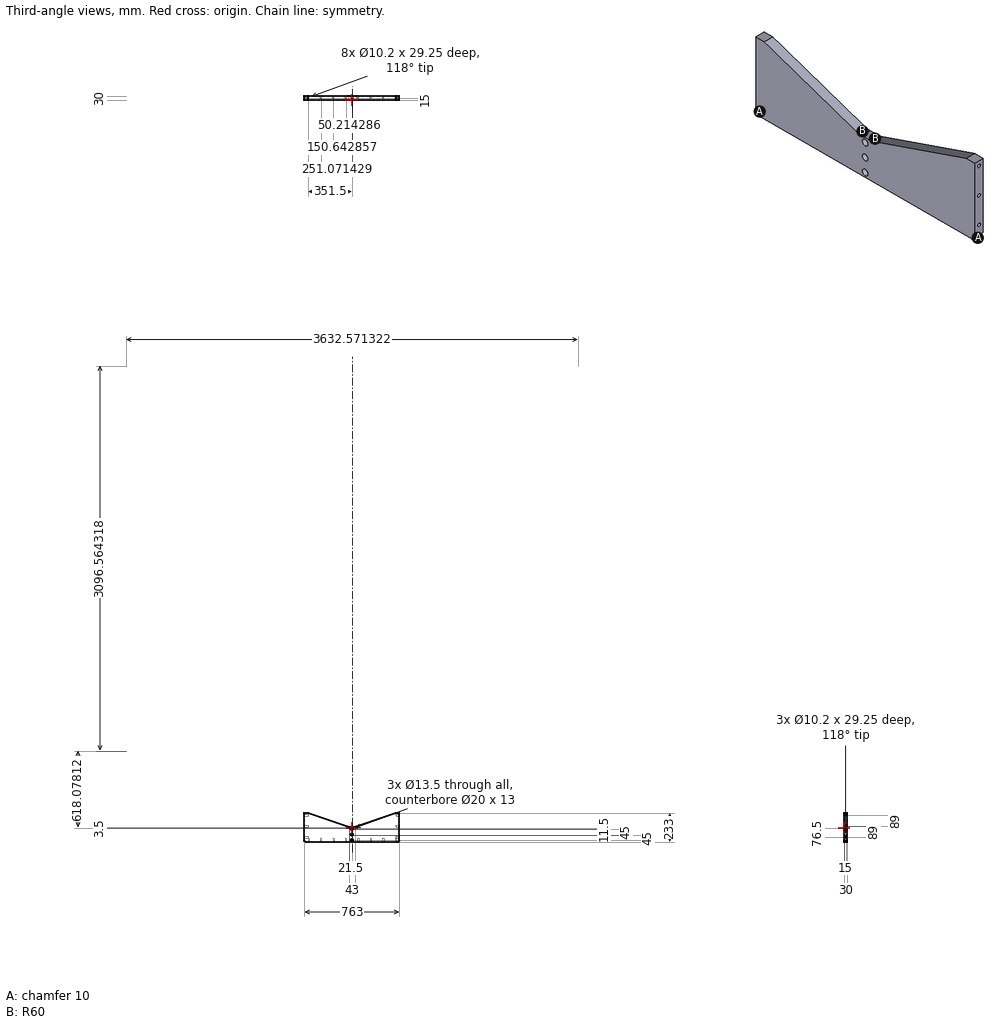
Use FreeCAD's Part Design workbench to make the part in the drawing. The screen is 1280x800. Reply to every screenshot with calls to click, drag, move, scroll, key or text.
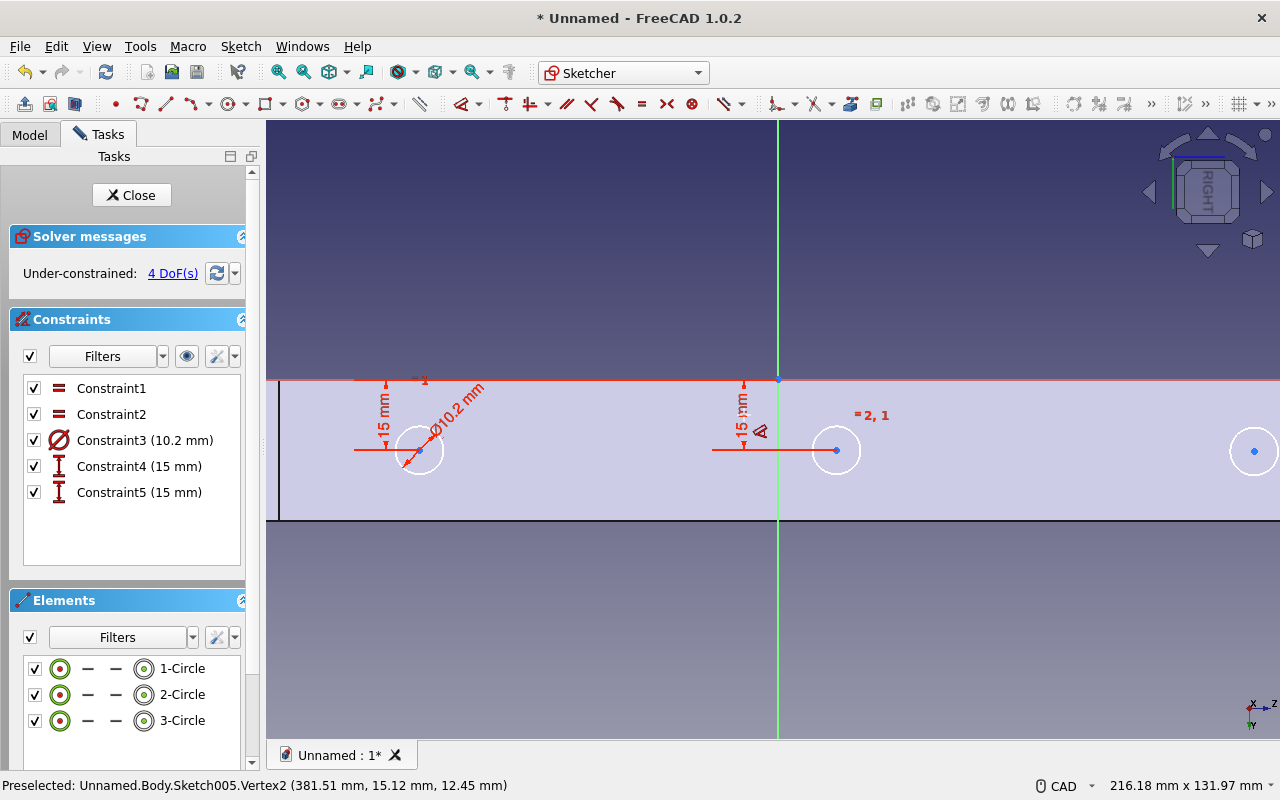
scroll(435, 434, down, 2)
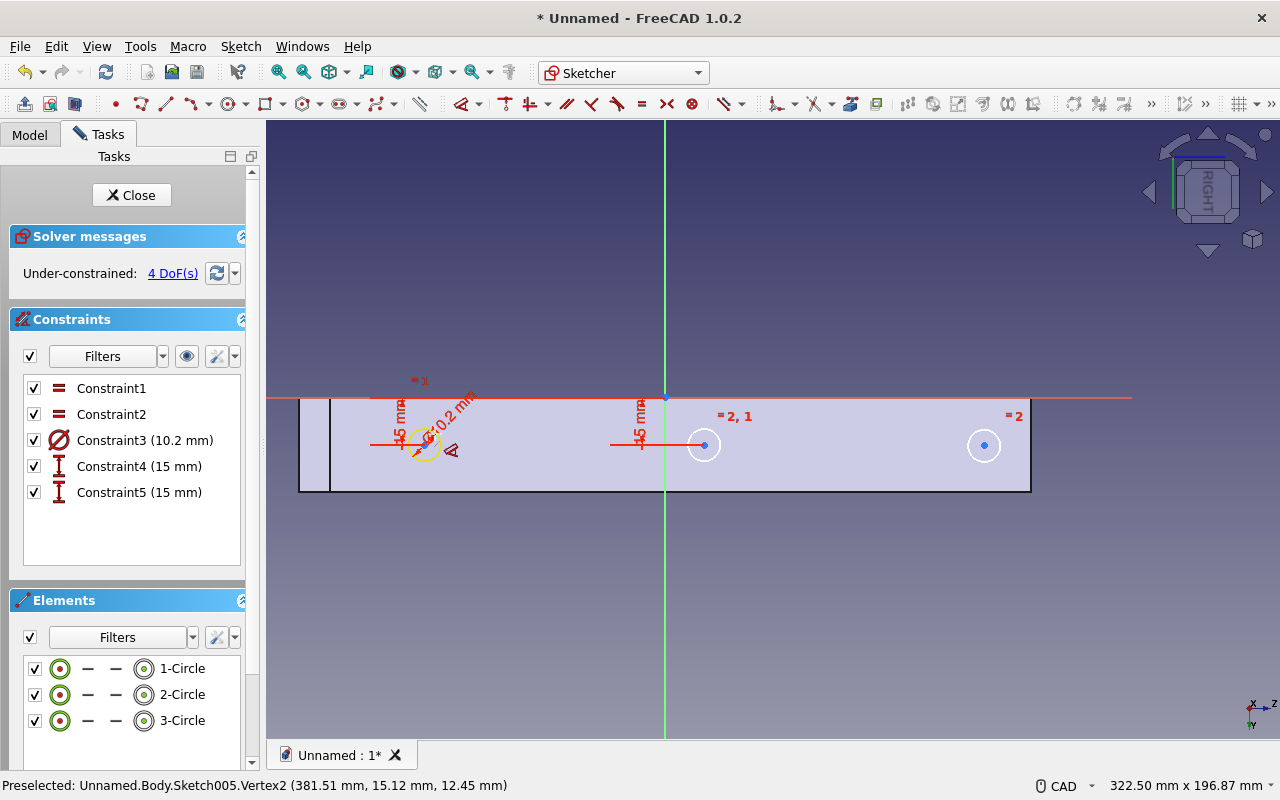
click(984, 446)
click(1018, 422)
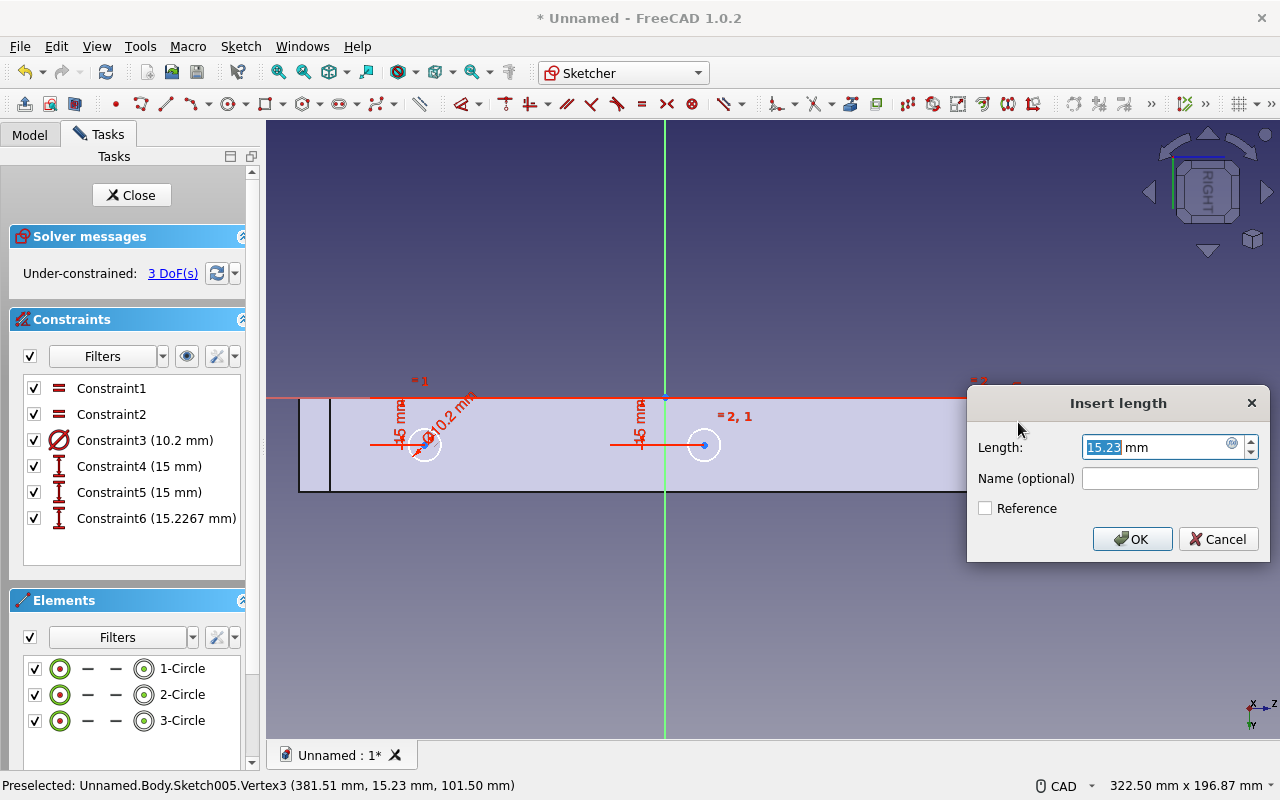
text(15)
key(Return)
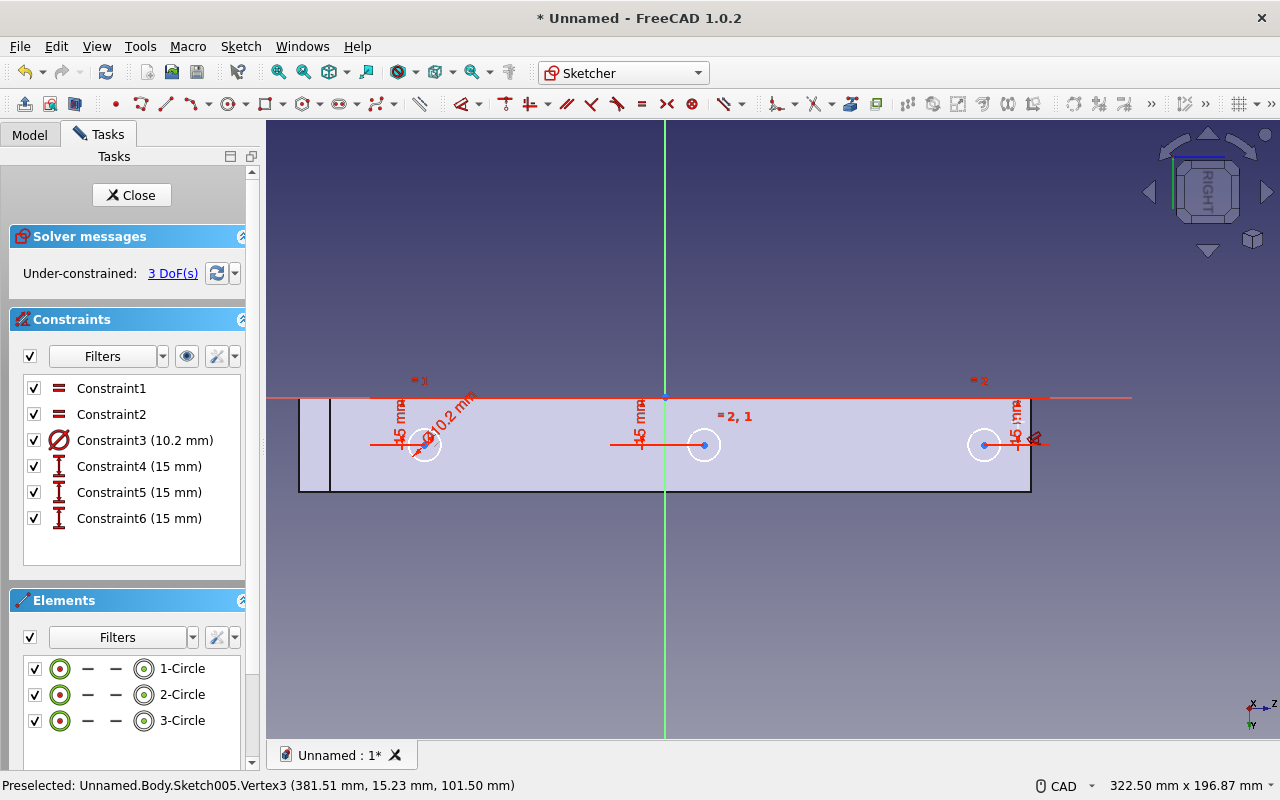
click(425, 445)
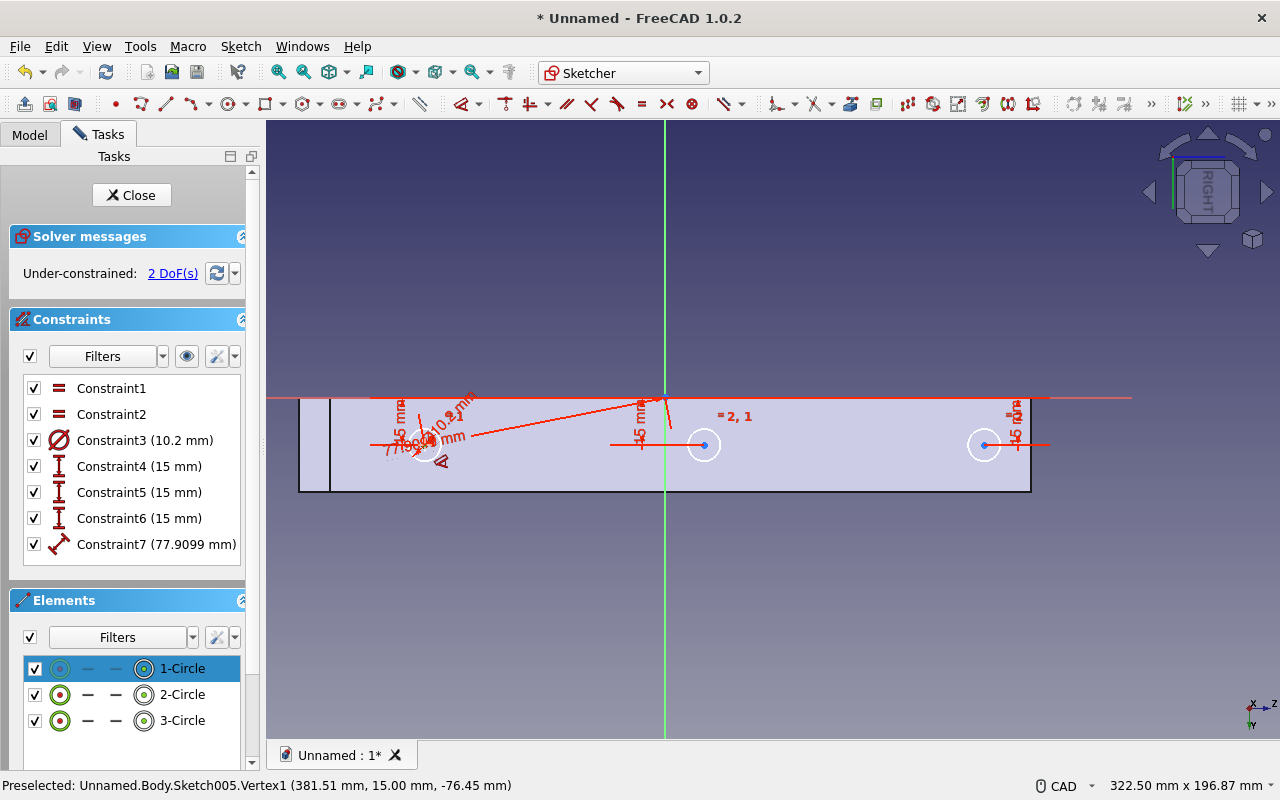
click(704, 445)
click(564, 479)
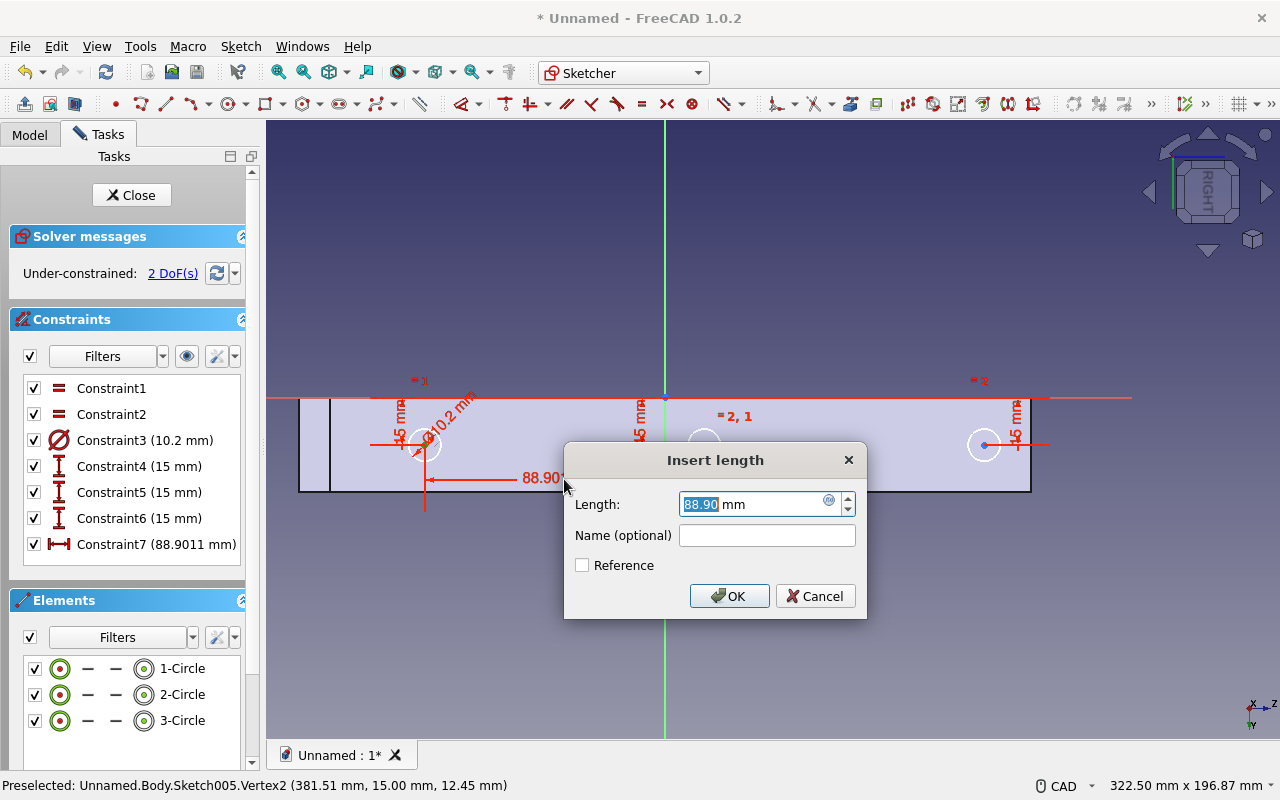
text(89)
key(Return)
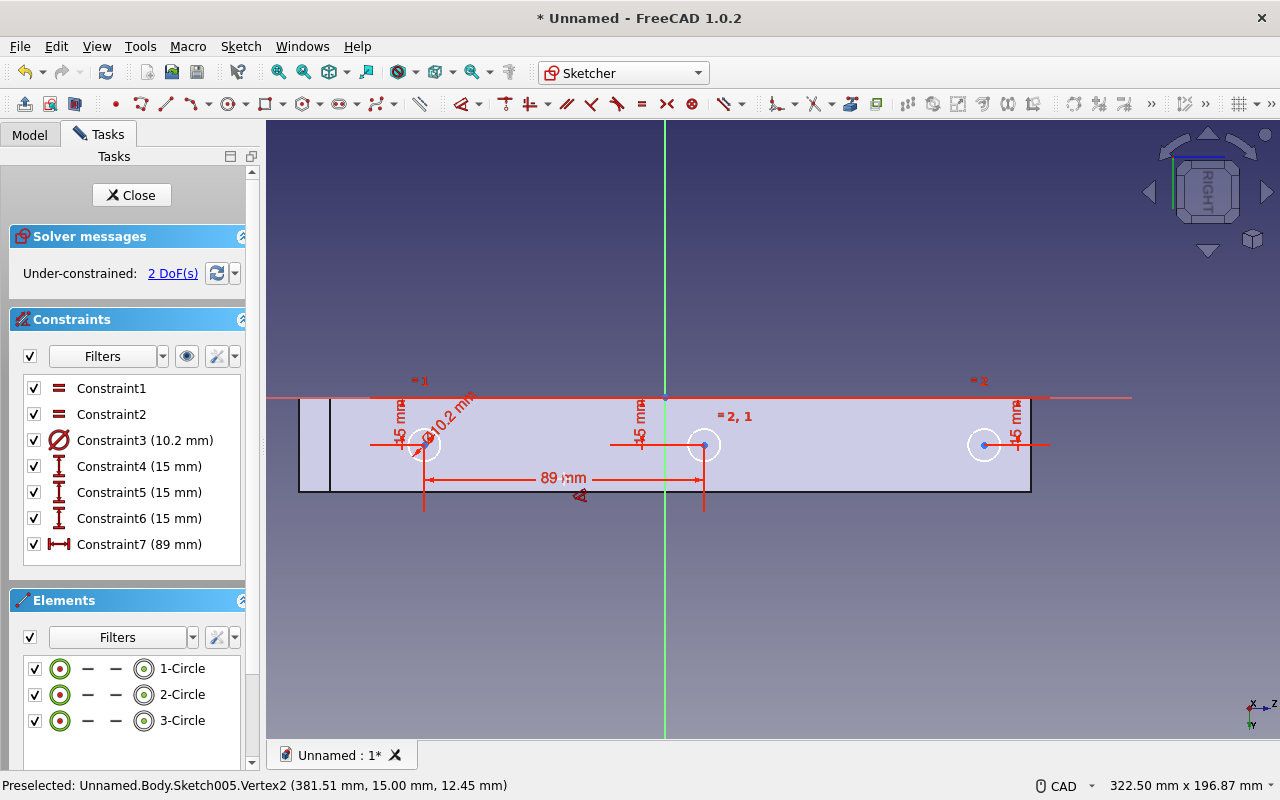
click(704, 445)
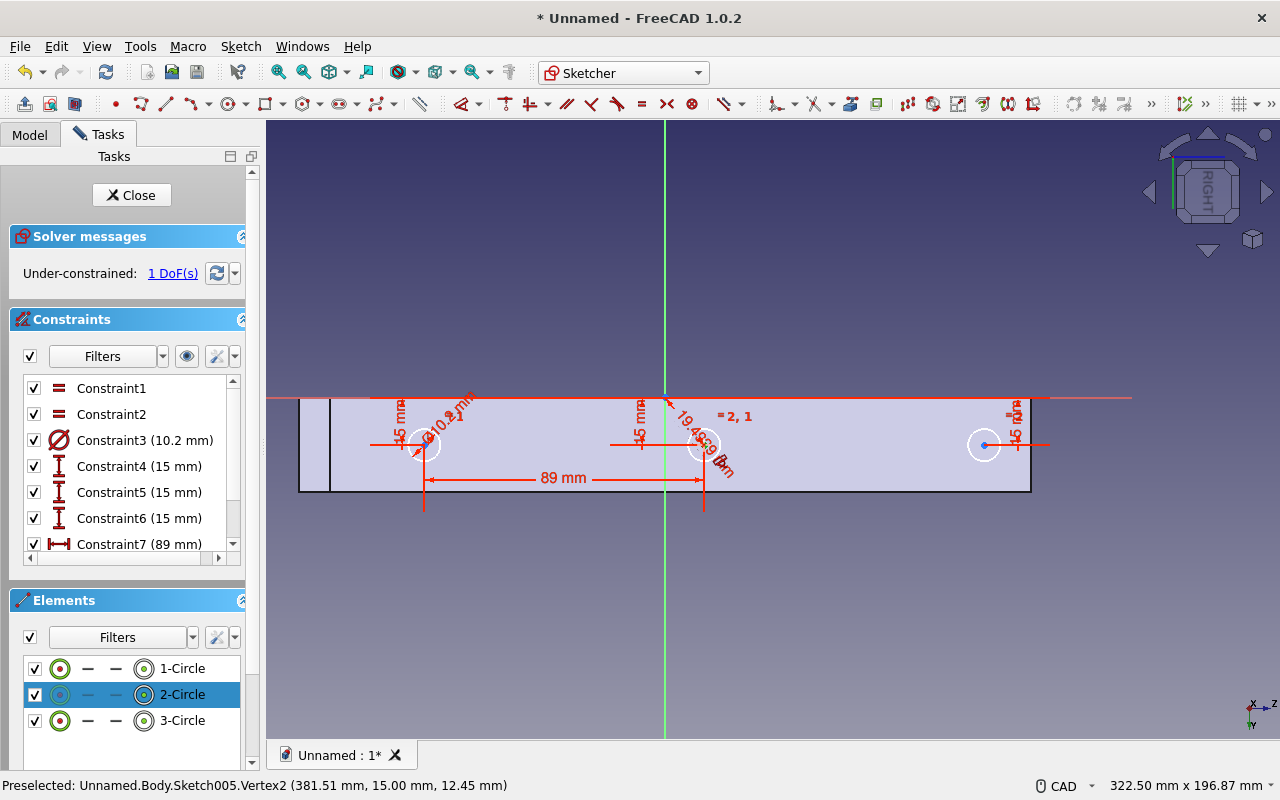
click(984, 445)
click(844, 479)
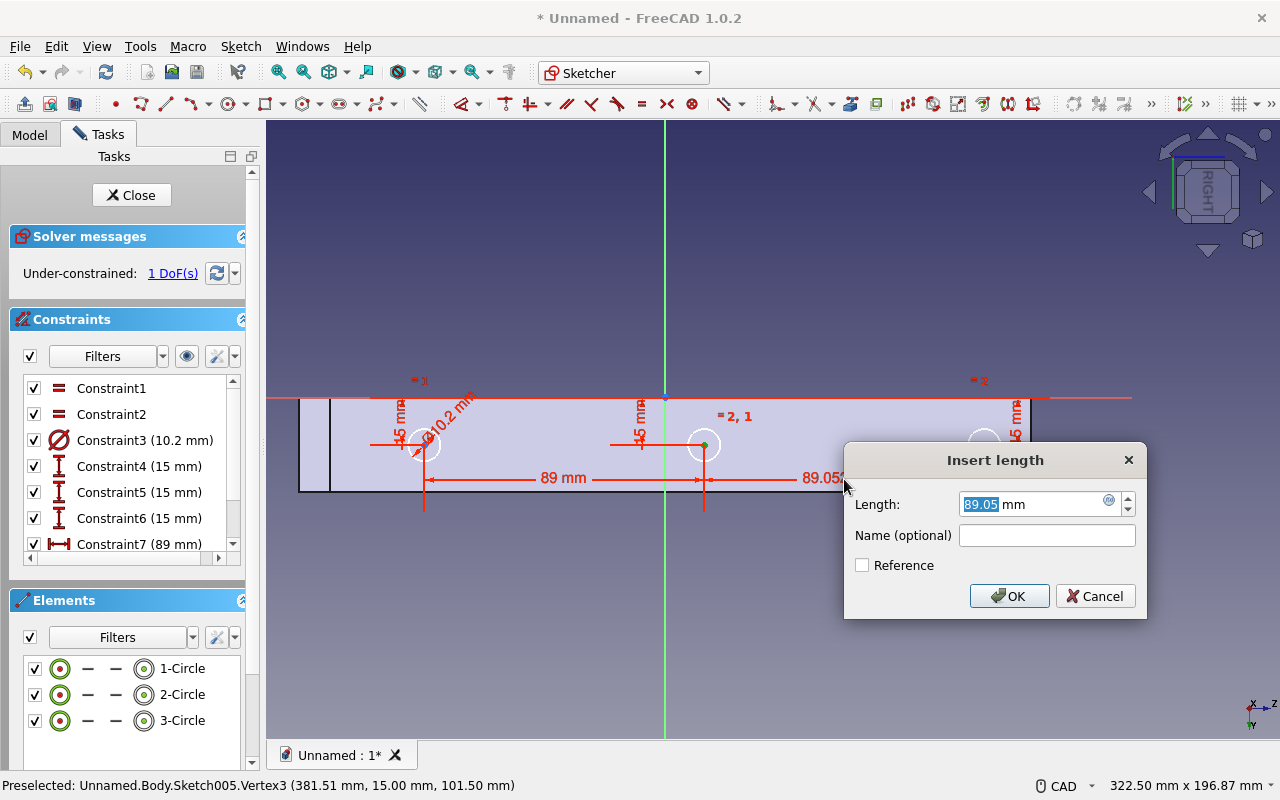
text(89)
key(Return)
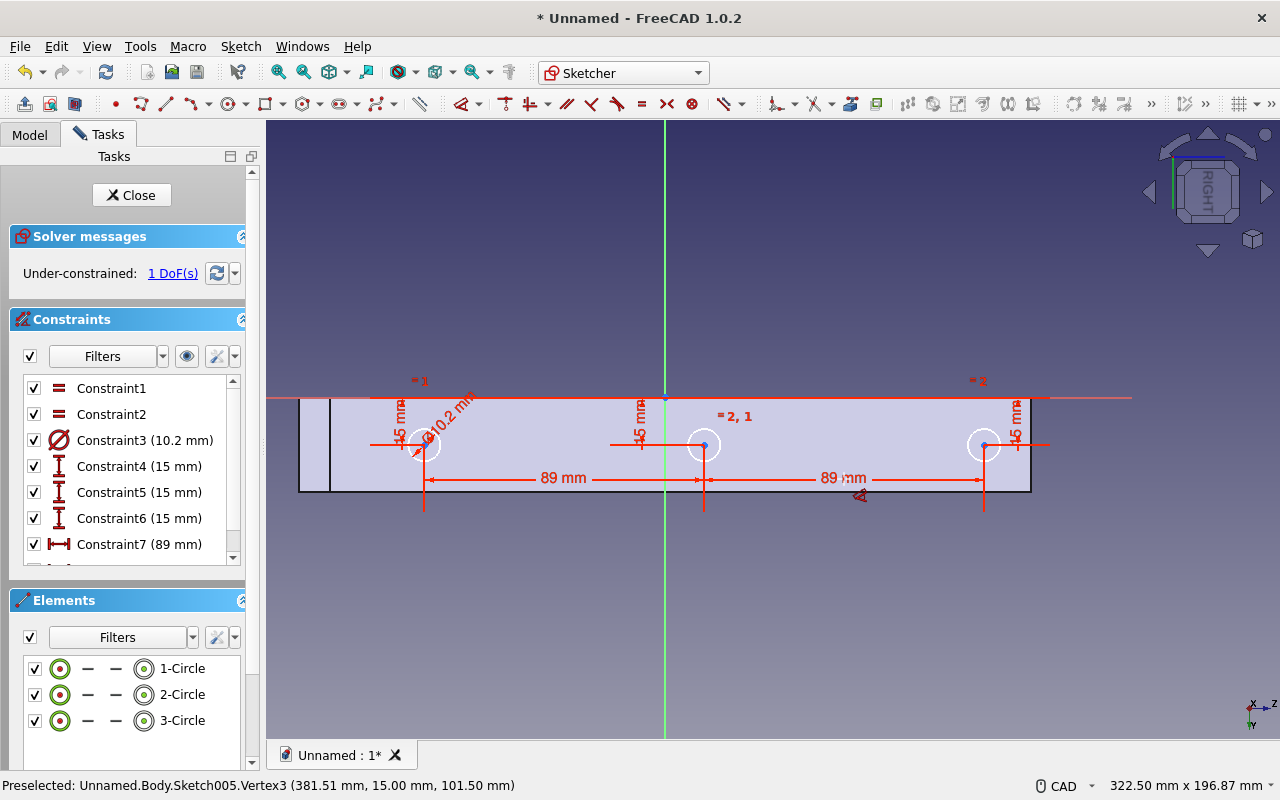
click(424, 445)
click(545, 364)